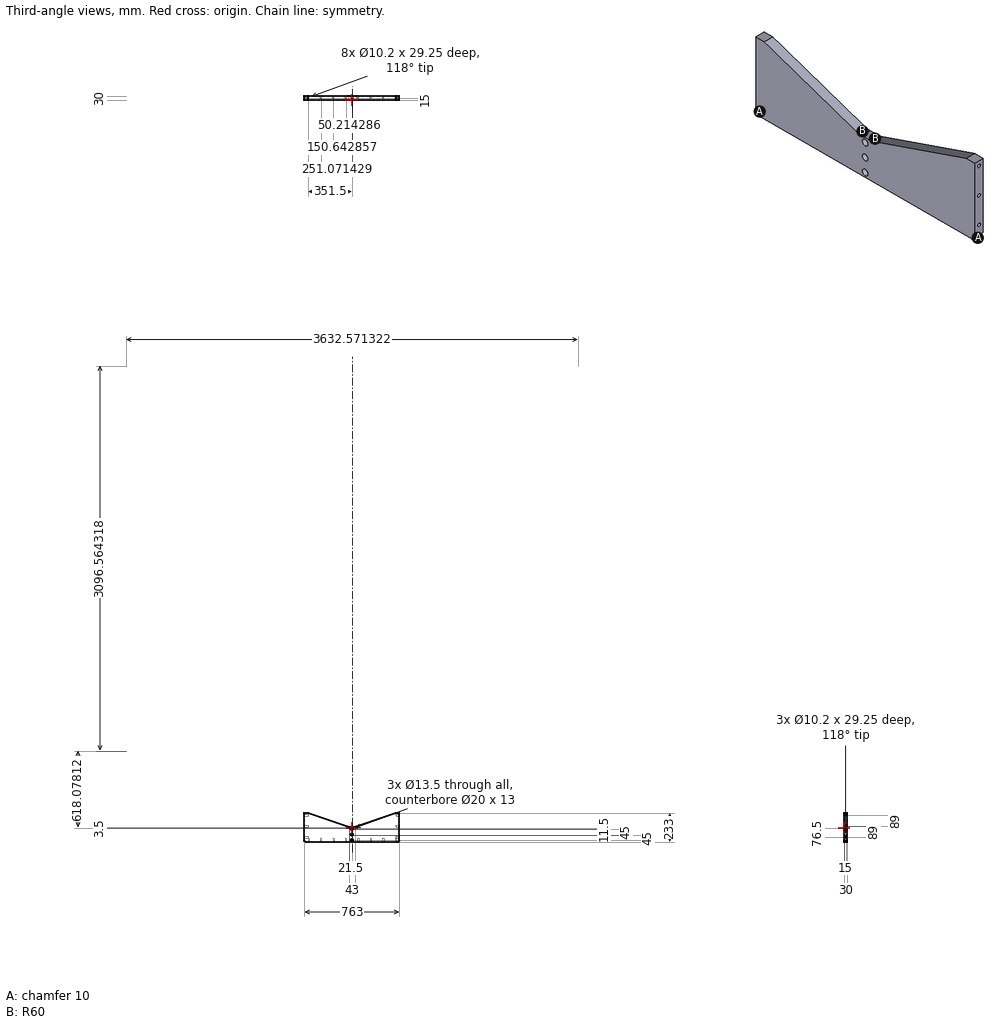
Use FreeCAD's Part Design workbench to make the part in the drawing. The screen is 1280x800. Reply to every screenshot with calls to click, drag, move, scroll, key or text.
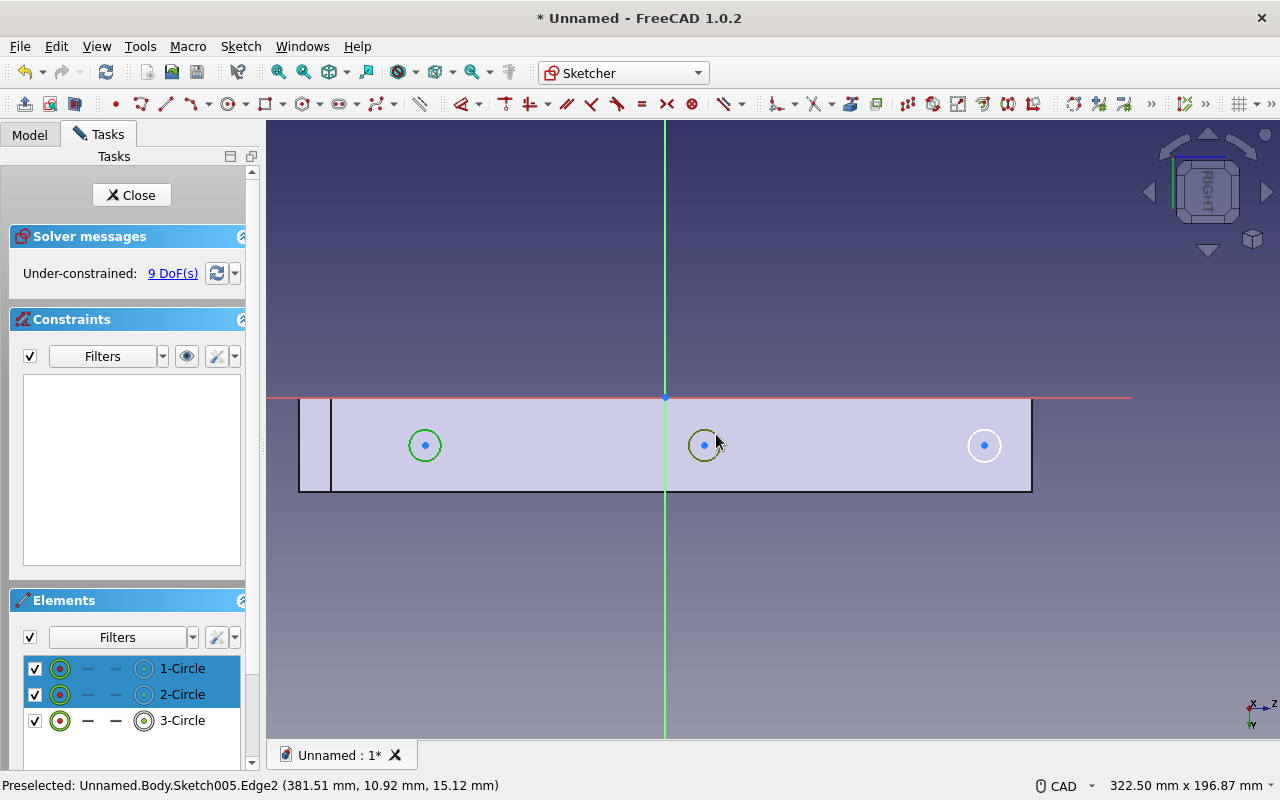
click(996, 434)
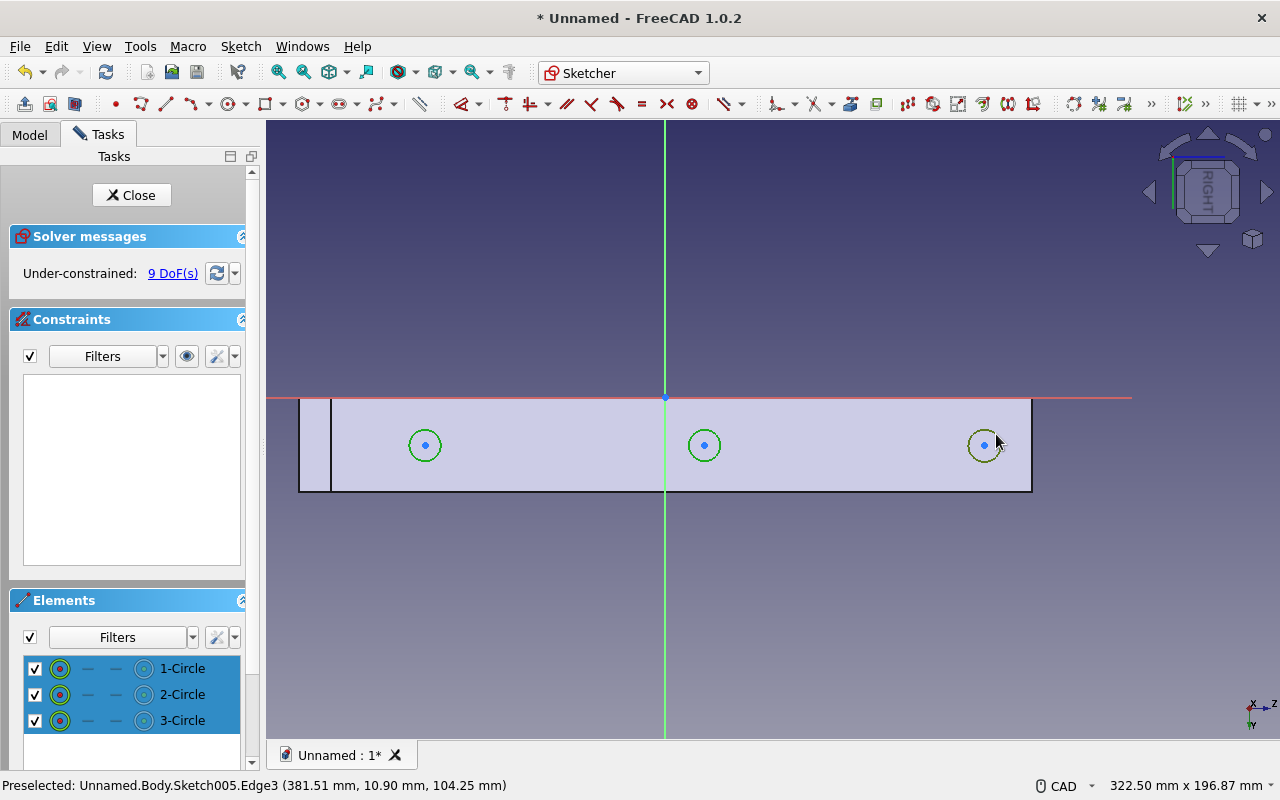
click(642, 104)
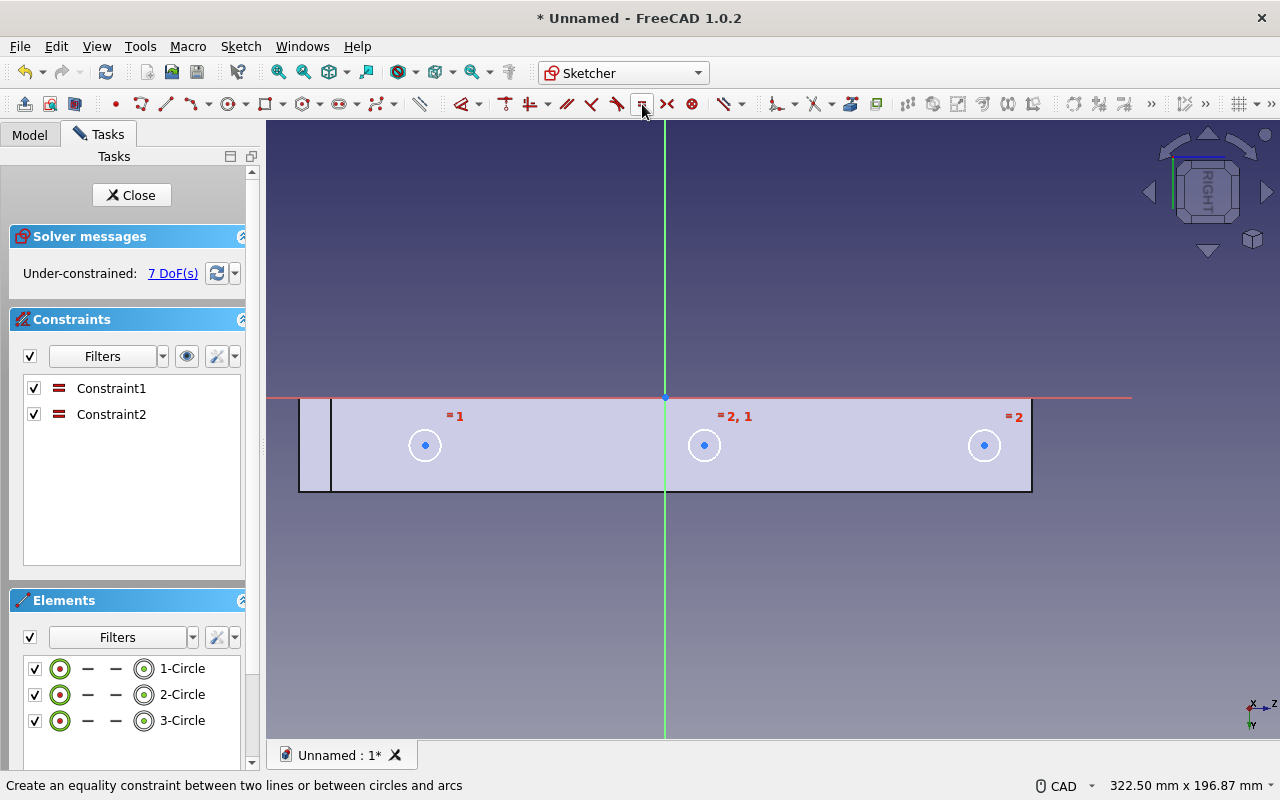
key(d)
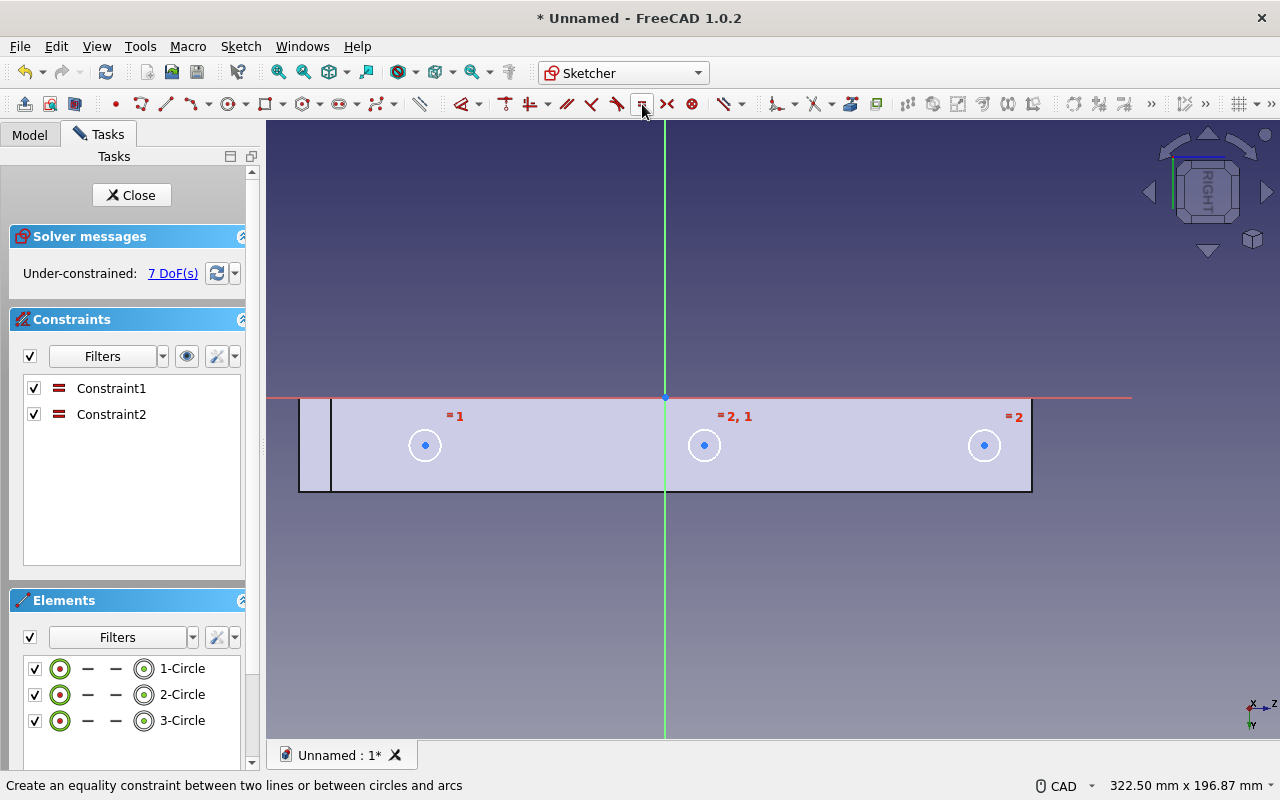
scroll(436, 434, up, 2)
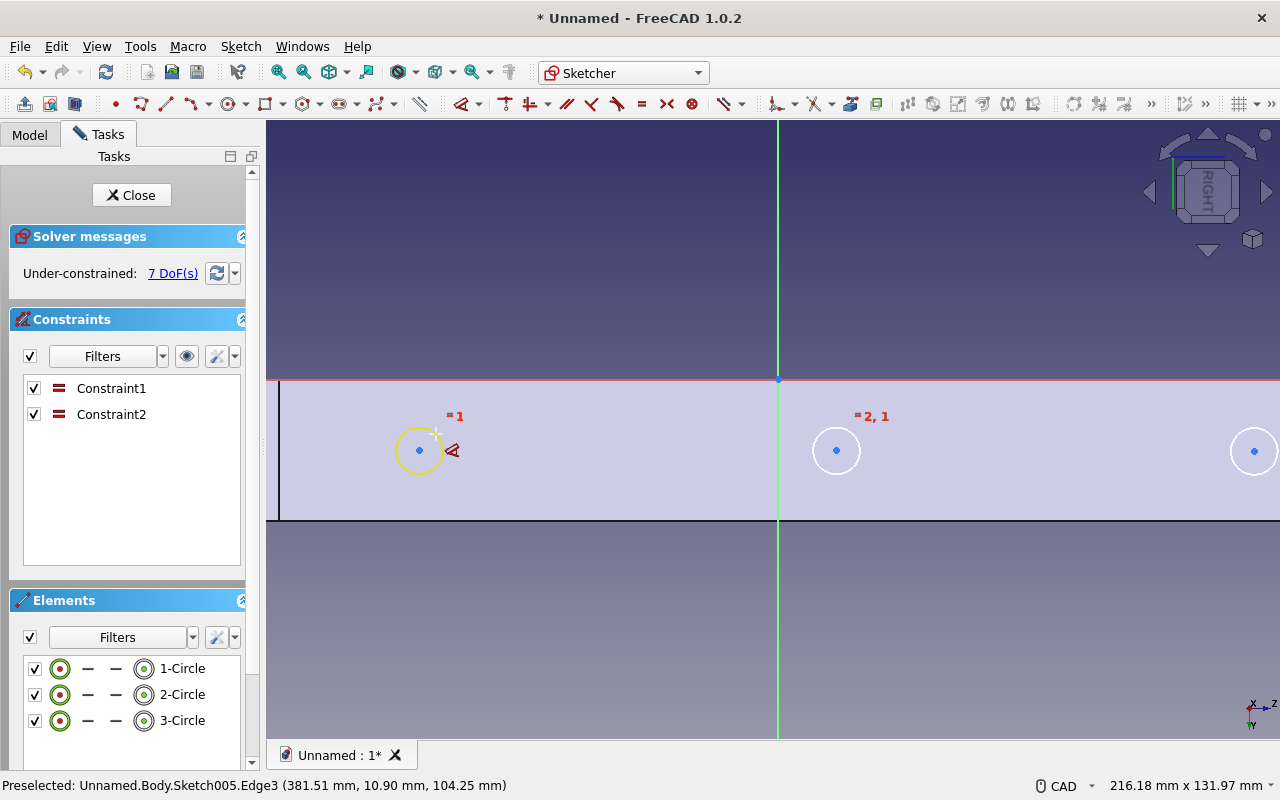
click(436, 434)
click(458, 411)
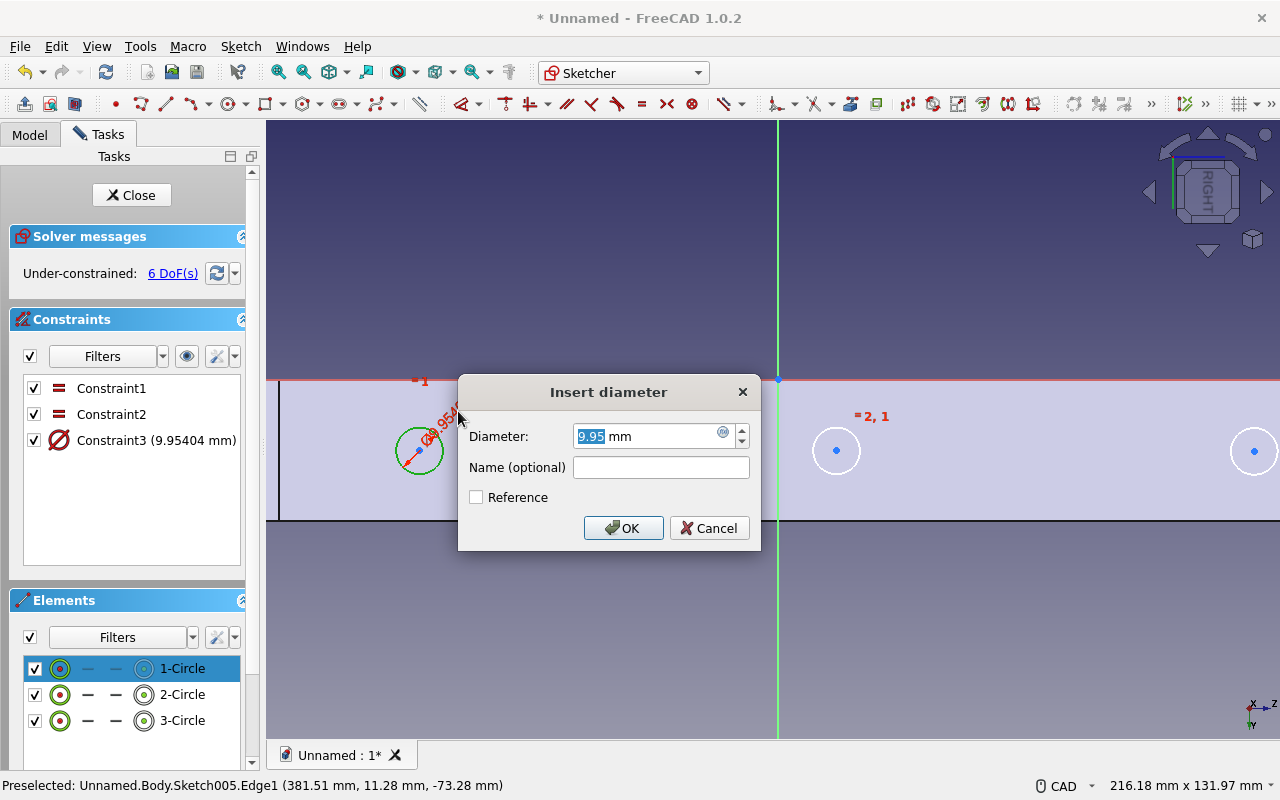
text(10.2)
key(Return)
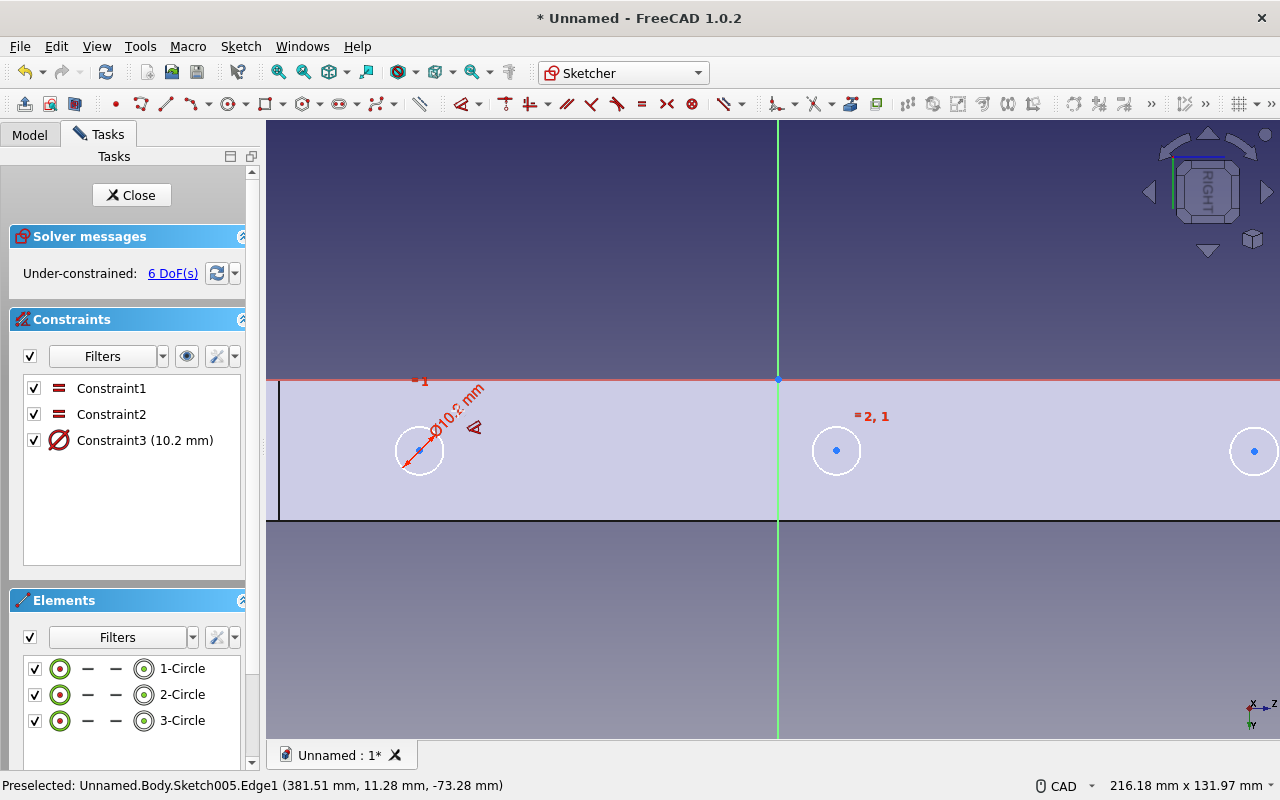
click(420, 451)
click(386, 415)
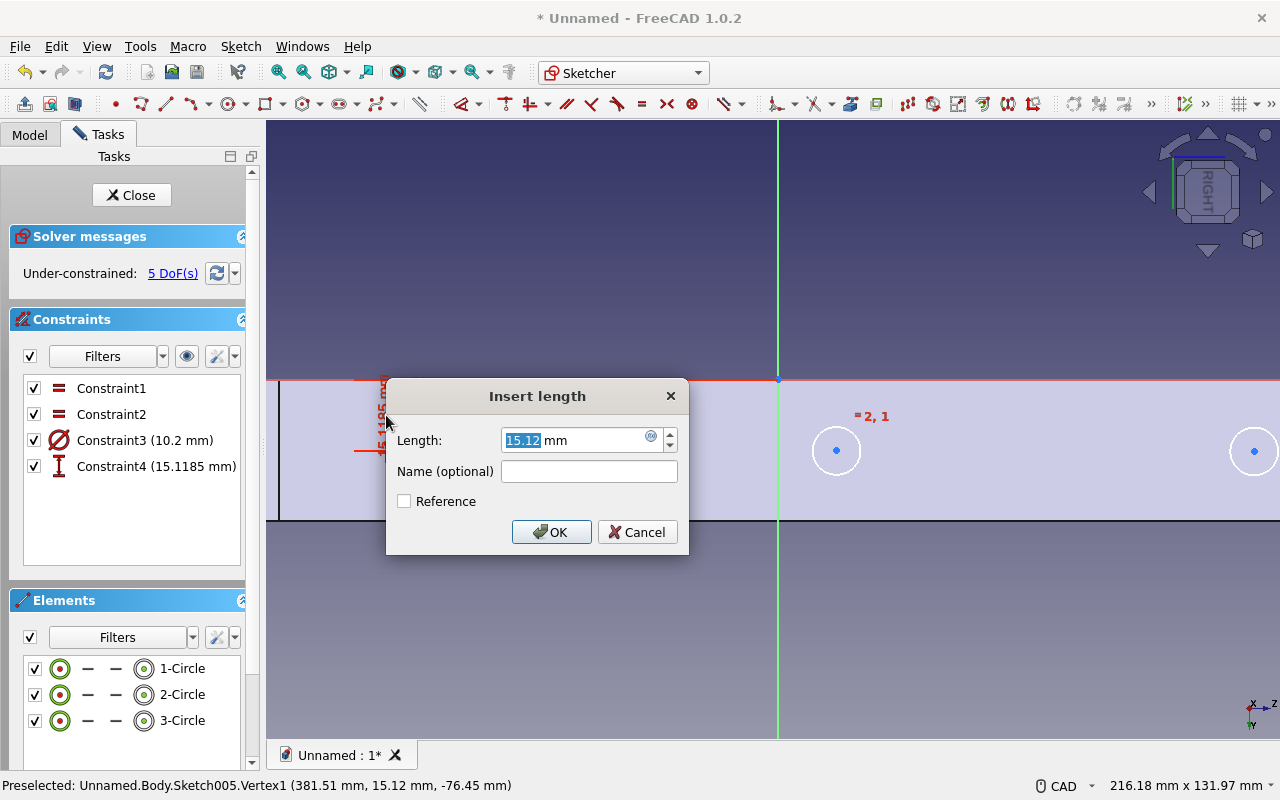
text(15)
key(Return)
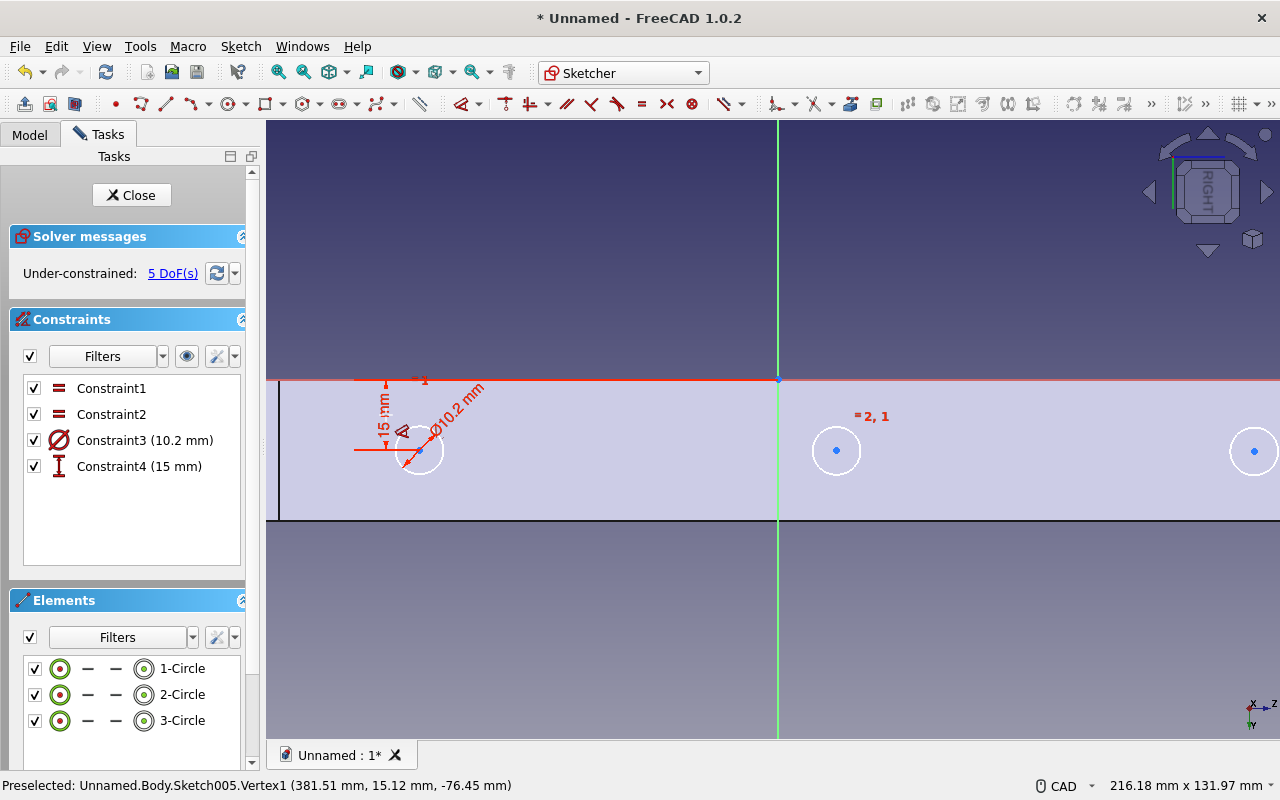
click(837, 451)
click(744, 415)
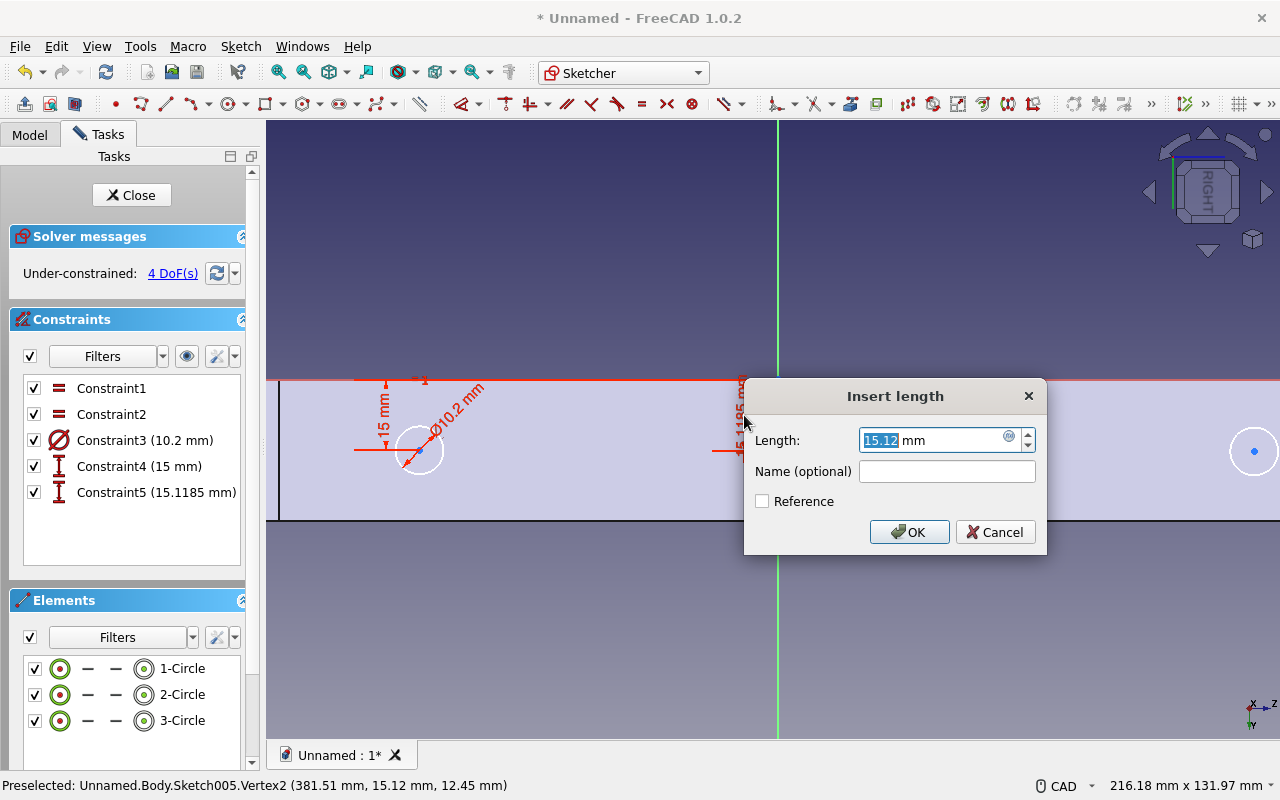
text(15)
key(Return)